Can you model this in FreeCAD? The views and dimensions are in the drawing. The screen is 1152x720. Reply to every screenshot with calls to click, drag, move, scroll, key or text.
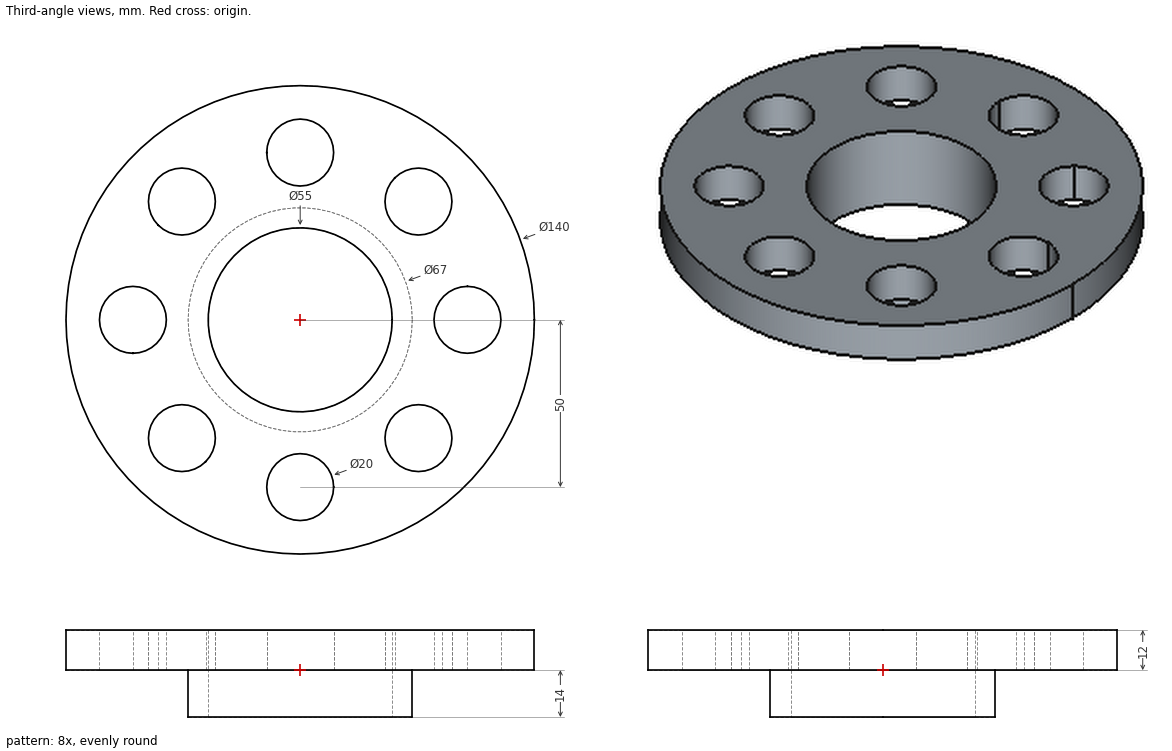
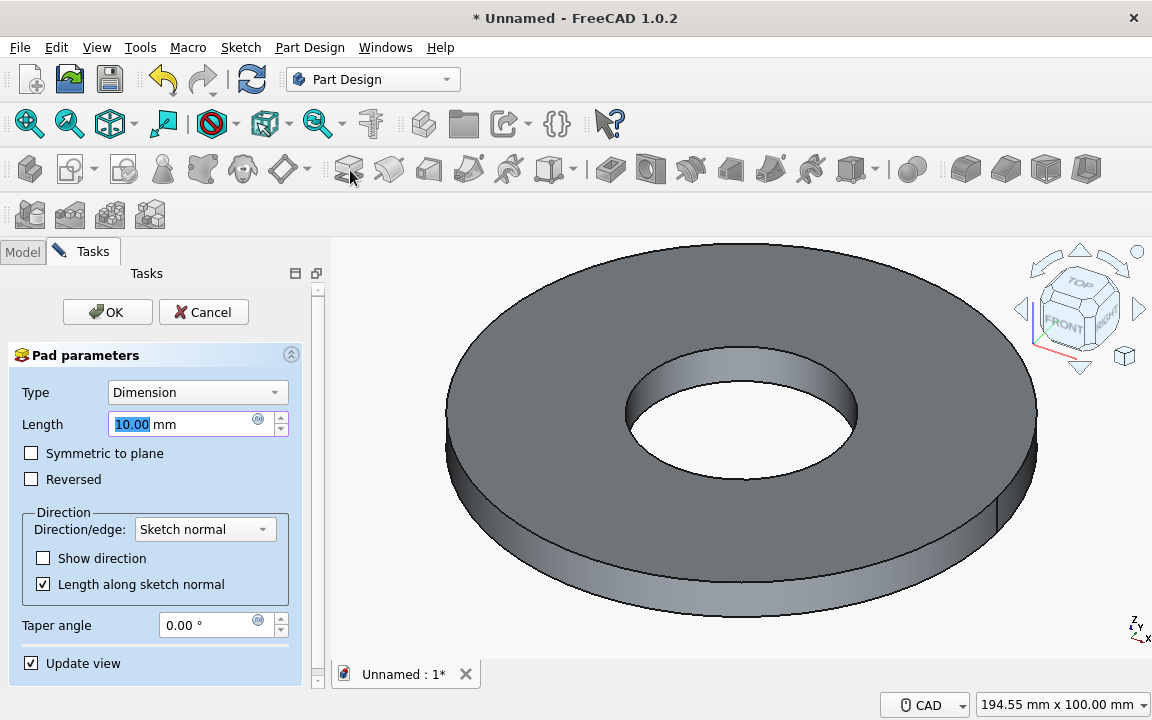
text(12)
key(Tab)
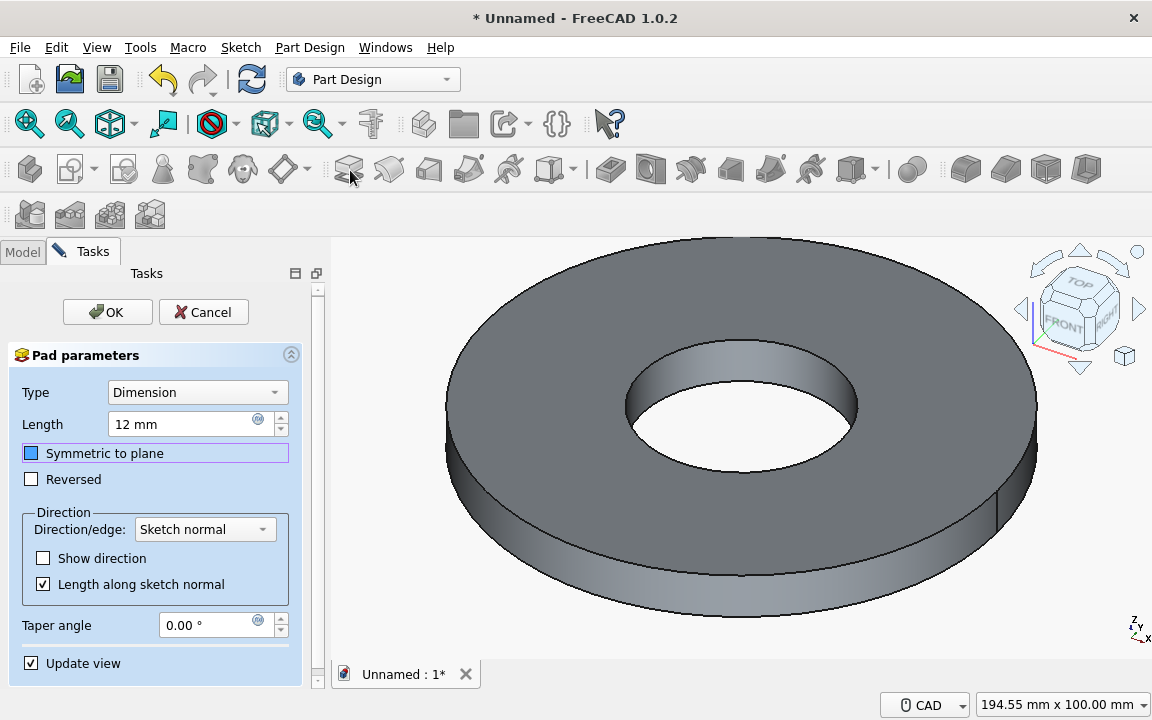
click(108, 312)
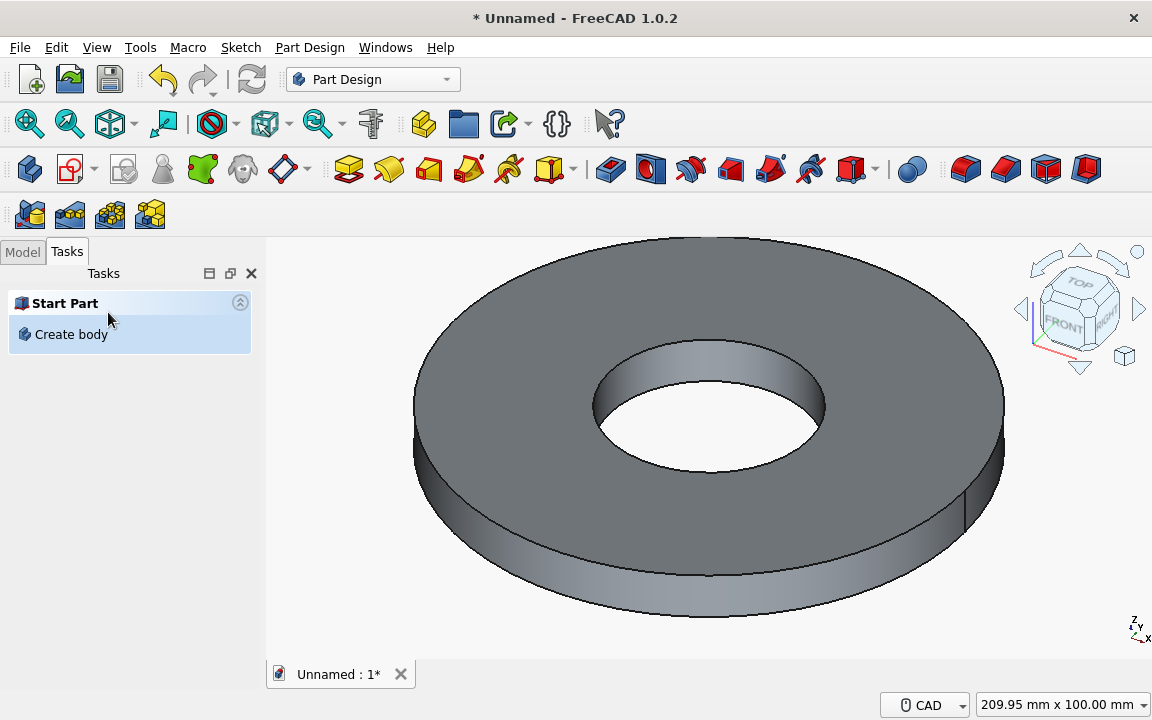
key(v)
key(f)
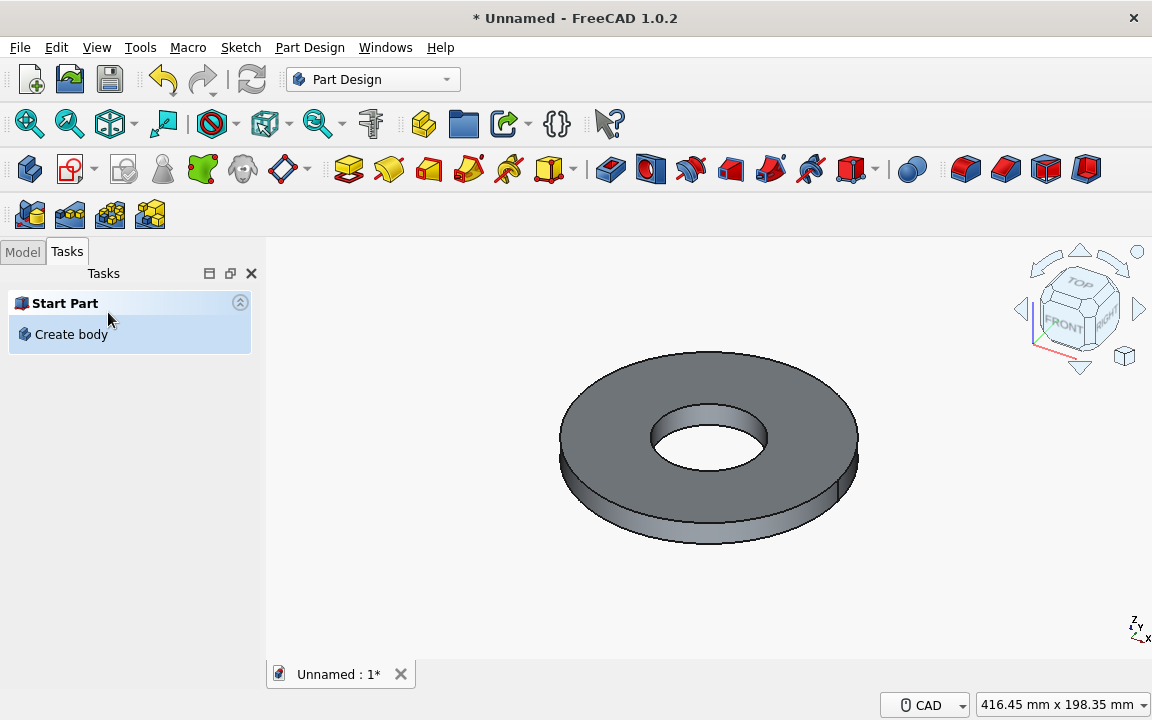
click(715, 382)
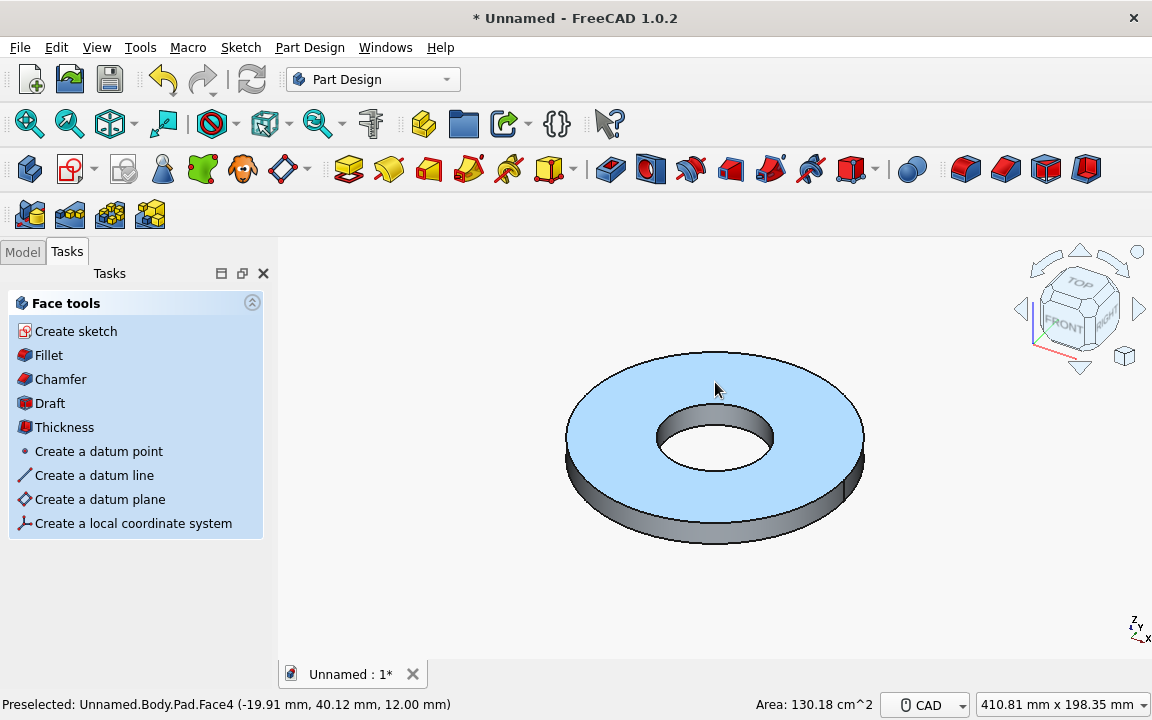
click(70, 170)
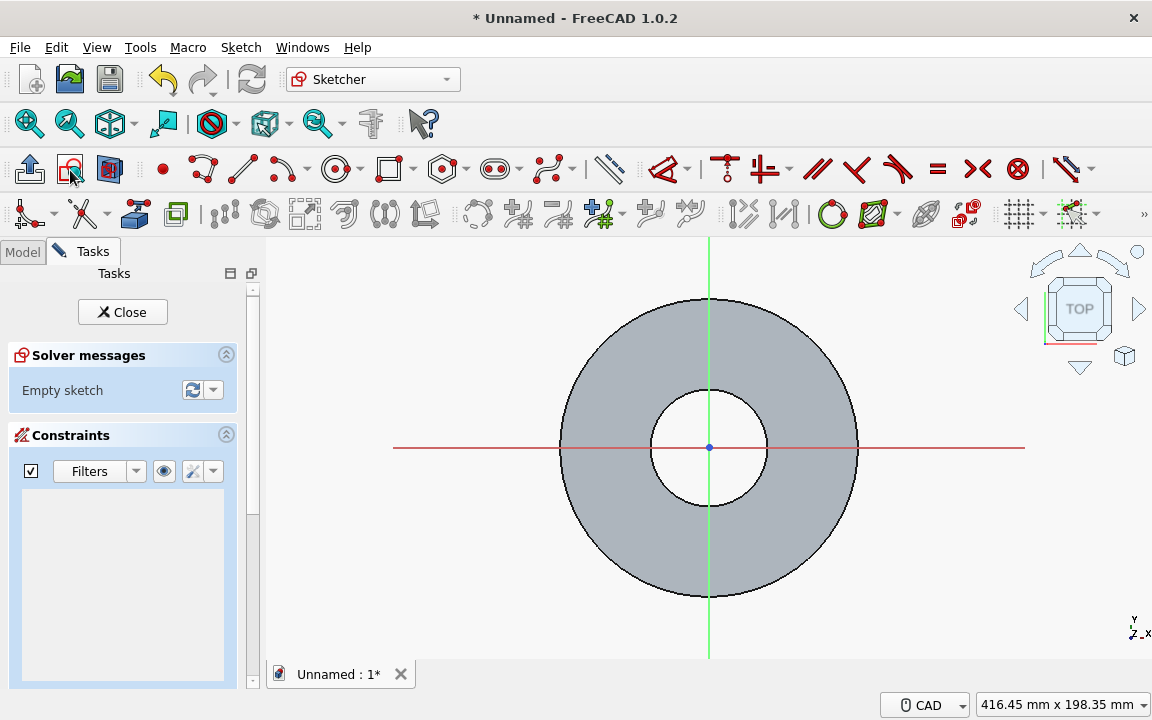
scroll(723, 575, up, 9)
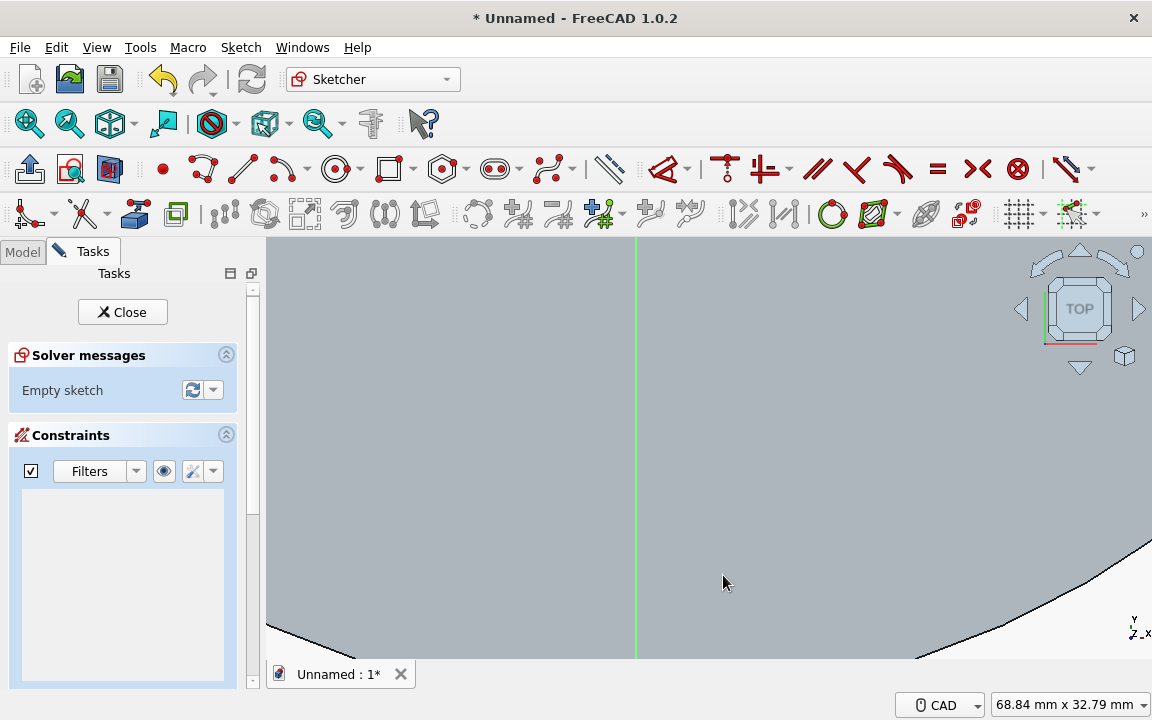
key(g)
key(c)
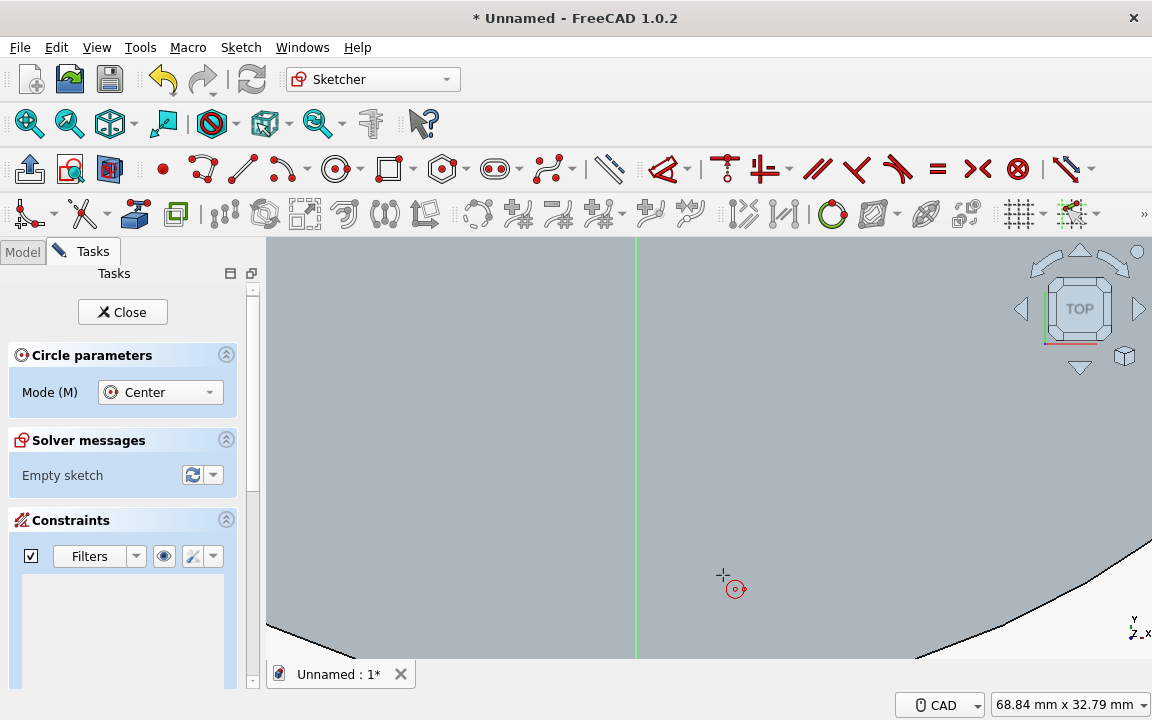
click(636, 446)
move(727, 355)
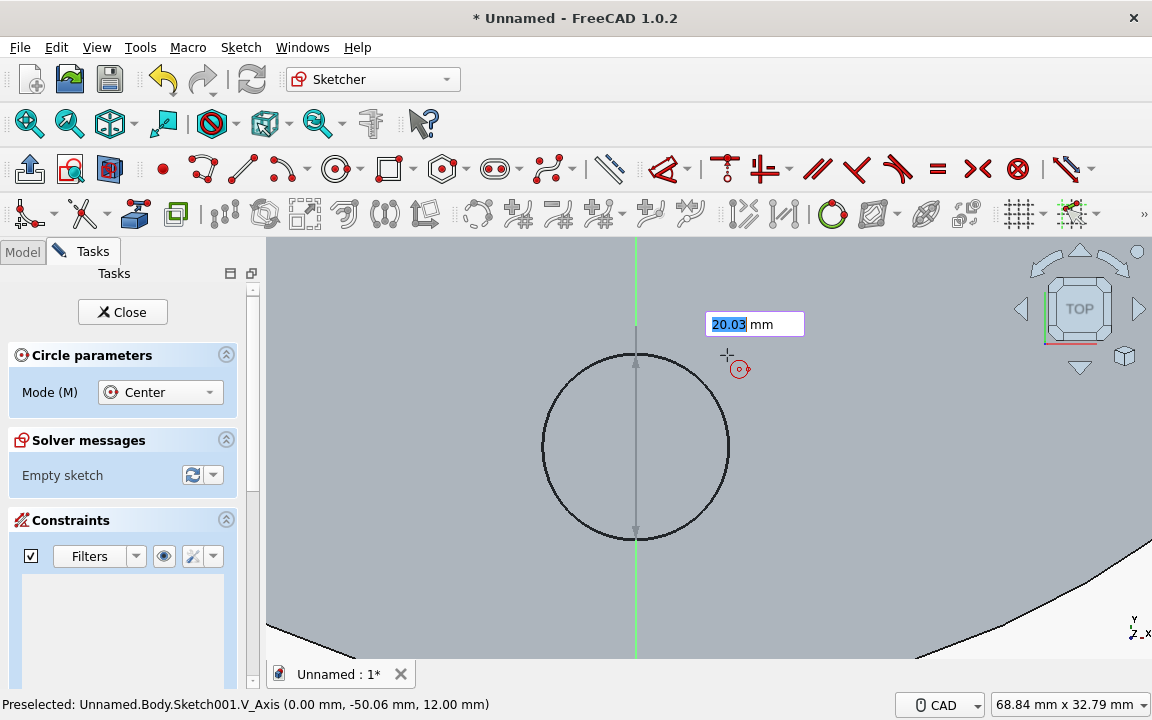
text(20)
key(Return)
key(Escape)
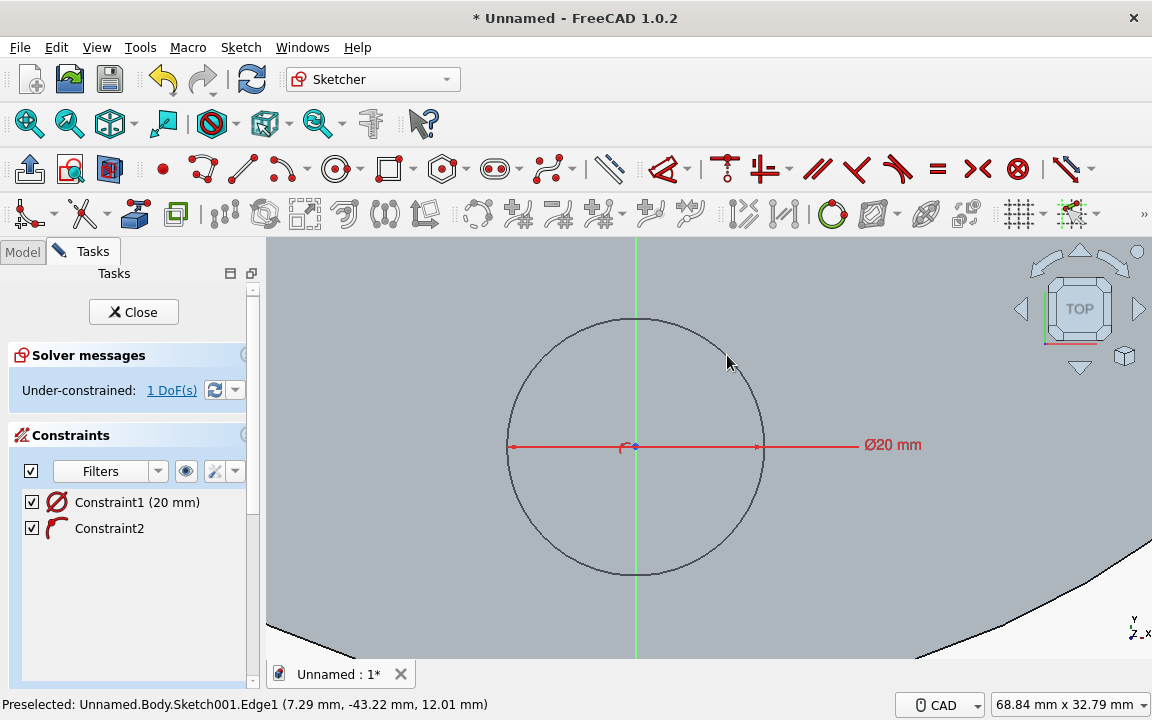
click(636, 447)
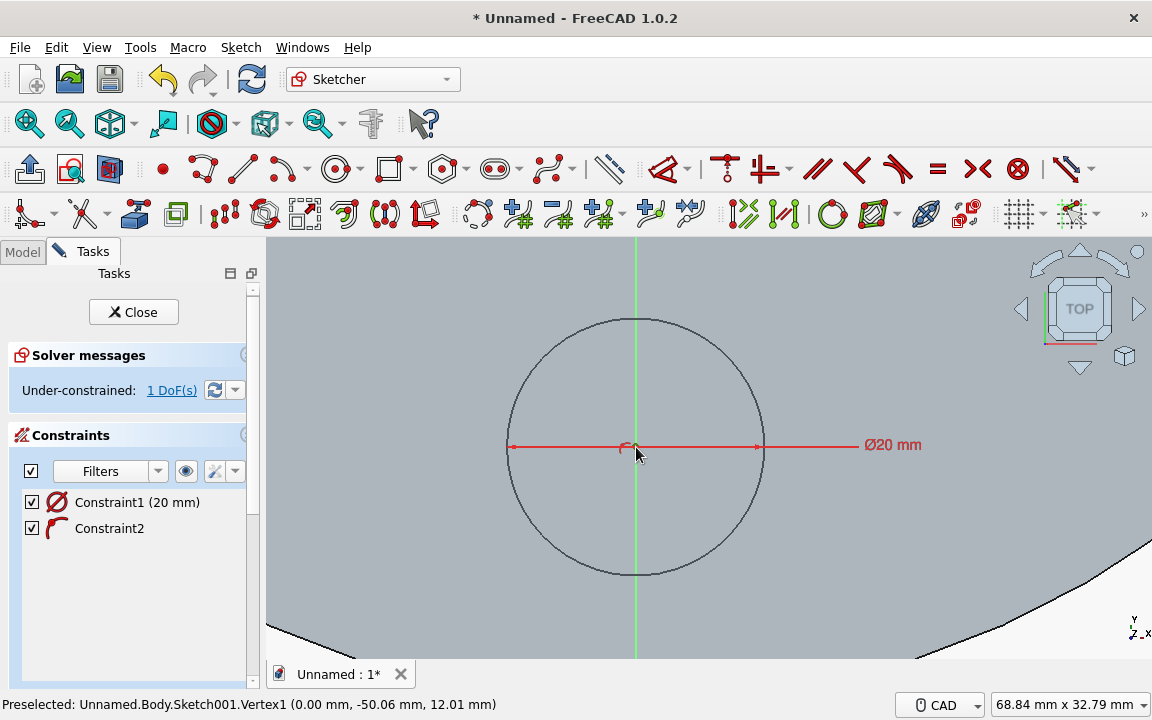
key(i)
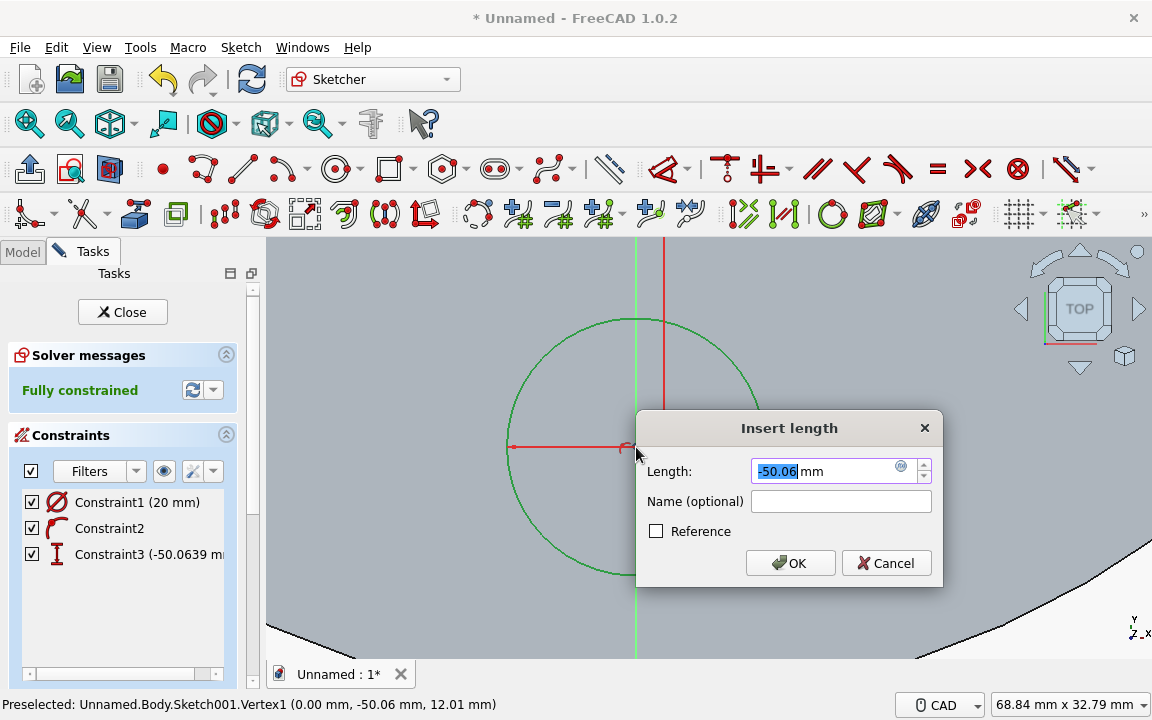
text(-50)
key(Return)